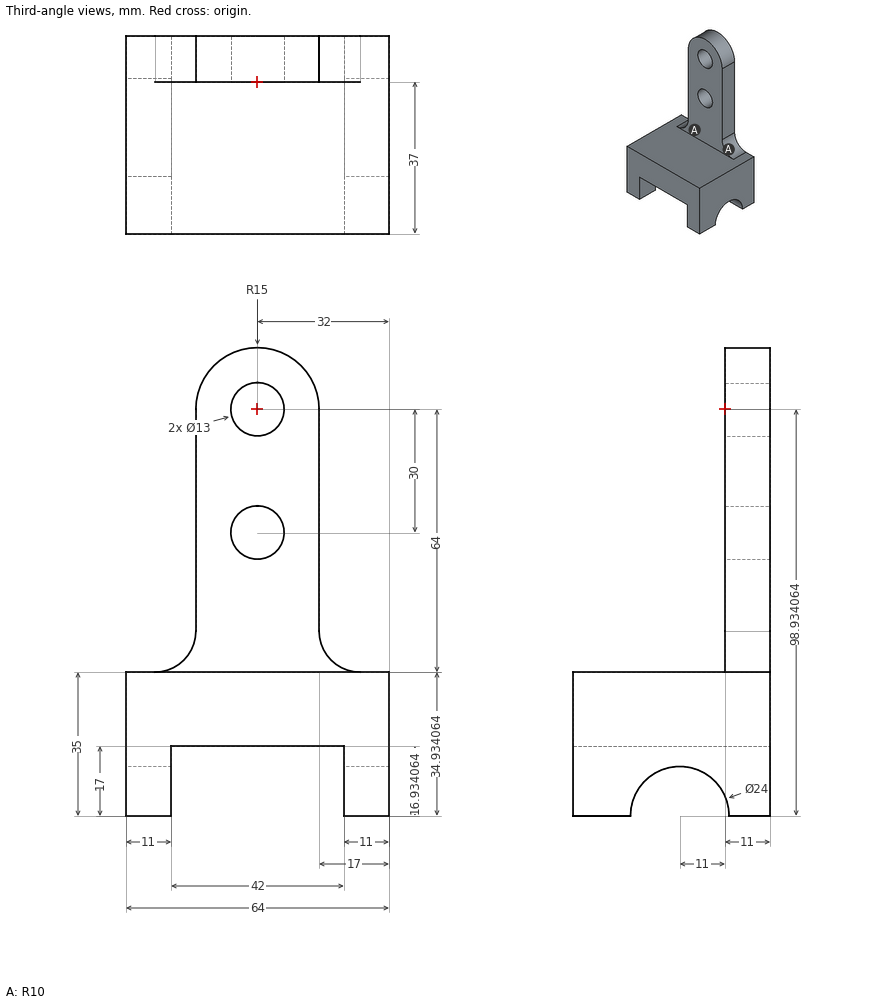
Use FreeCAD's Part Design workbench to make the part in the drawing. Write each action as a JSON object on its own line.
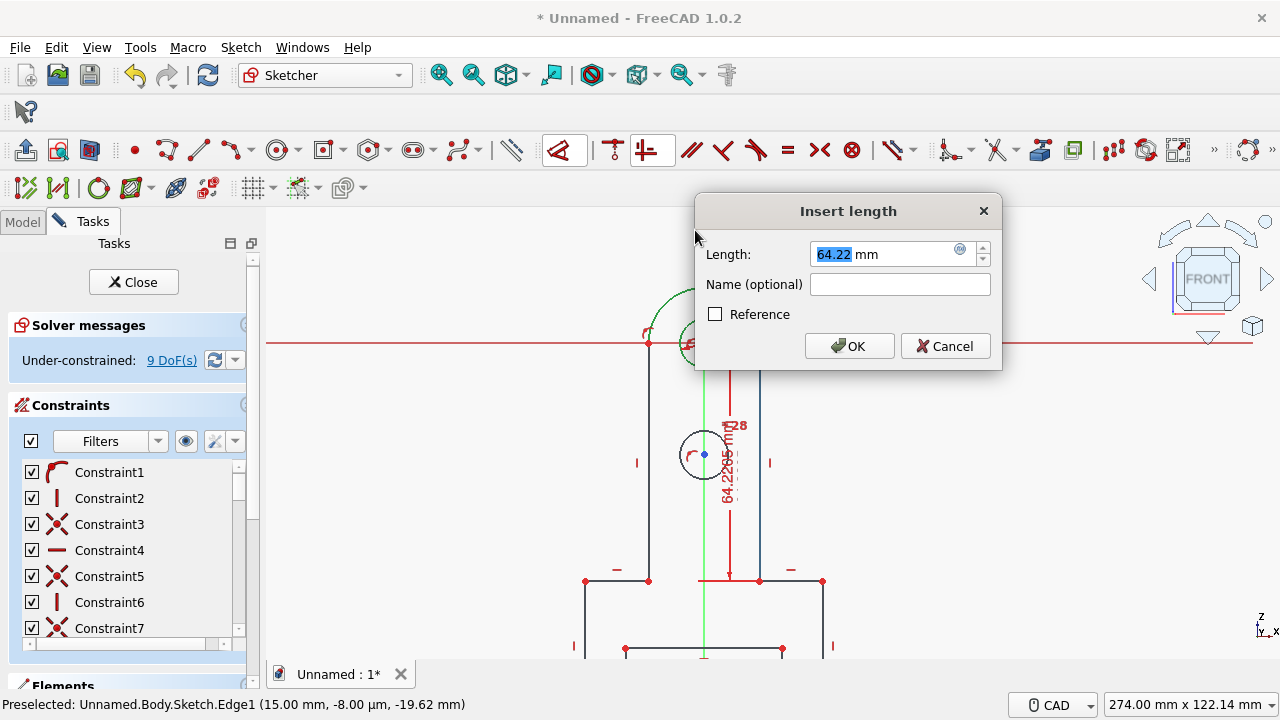
{"action": "type", "text": "64"}
{"action": "key", "text": "Return"}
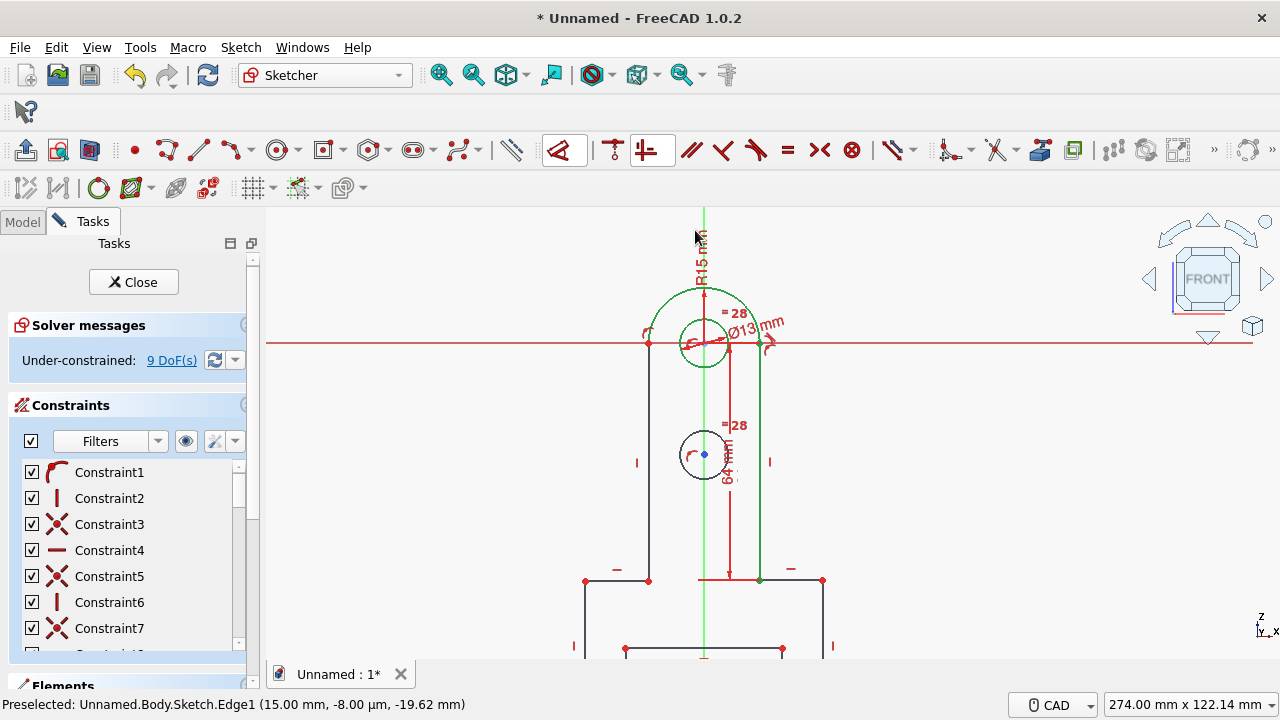
{"action": "left_click", "coordinate": [779, 580]}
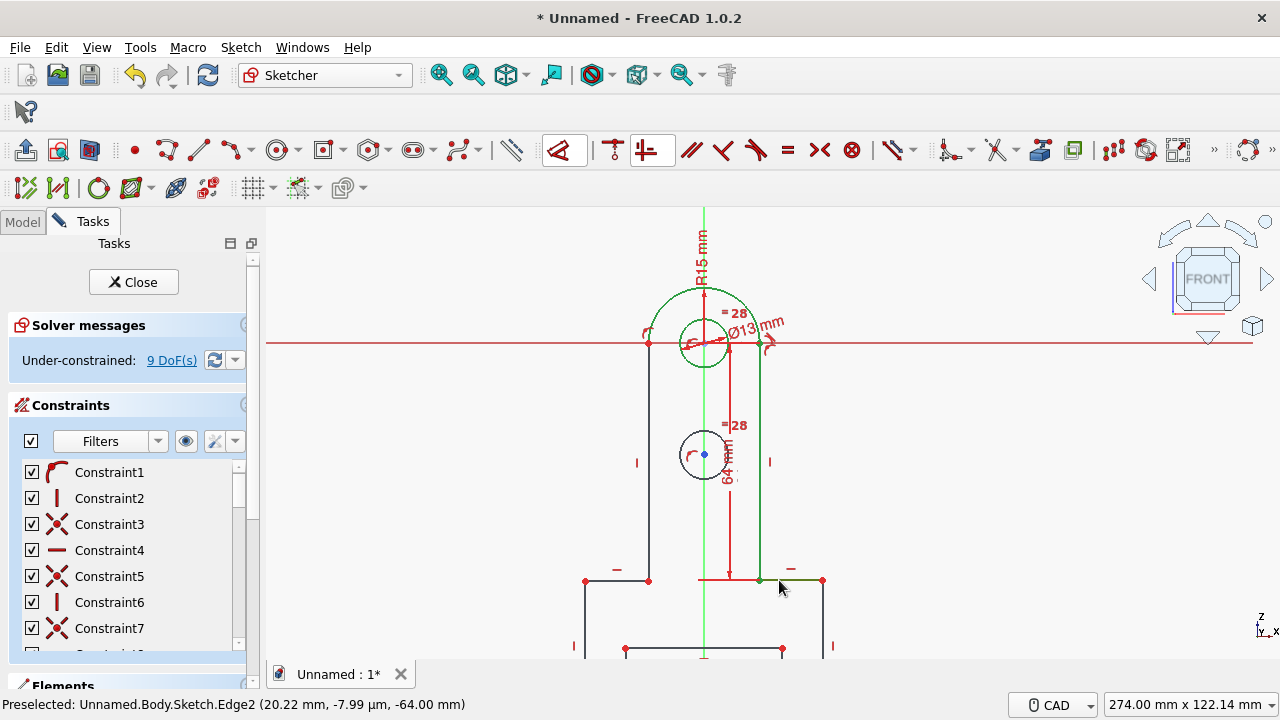
{"action": "left_click", "coordinate": [582, 150]}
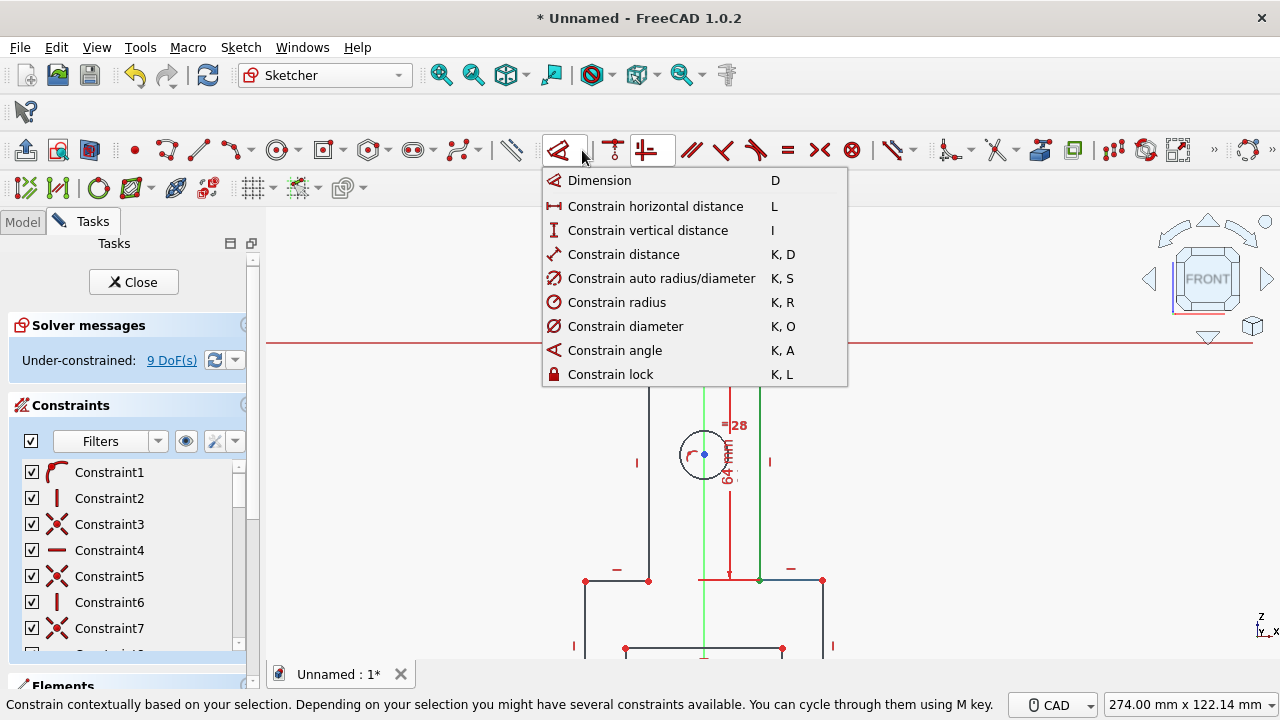
{"action": "left_click", "coordinate": [695, 206]}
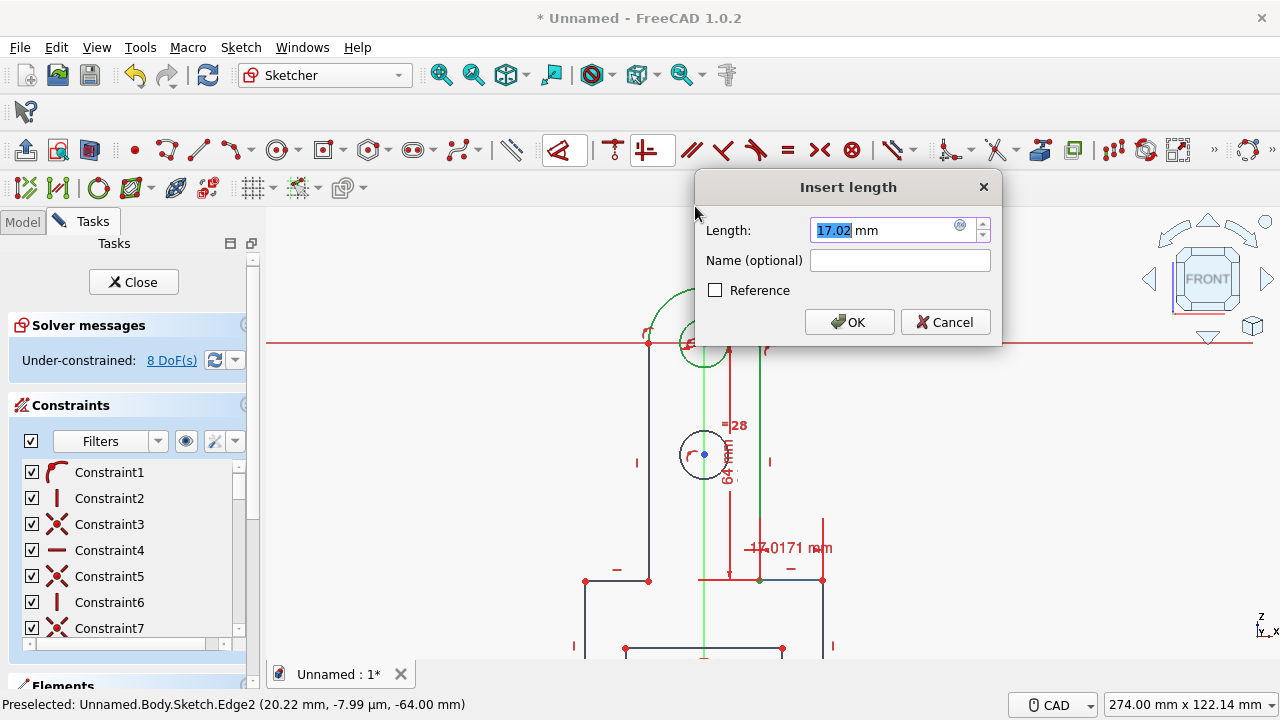
{"action": "type", "text": "17"}
{"action": "key", "text": "Return"}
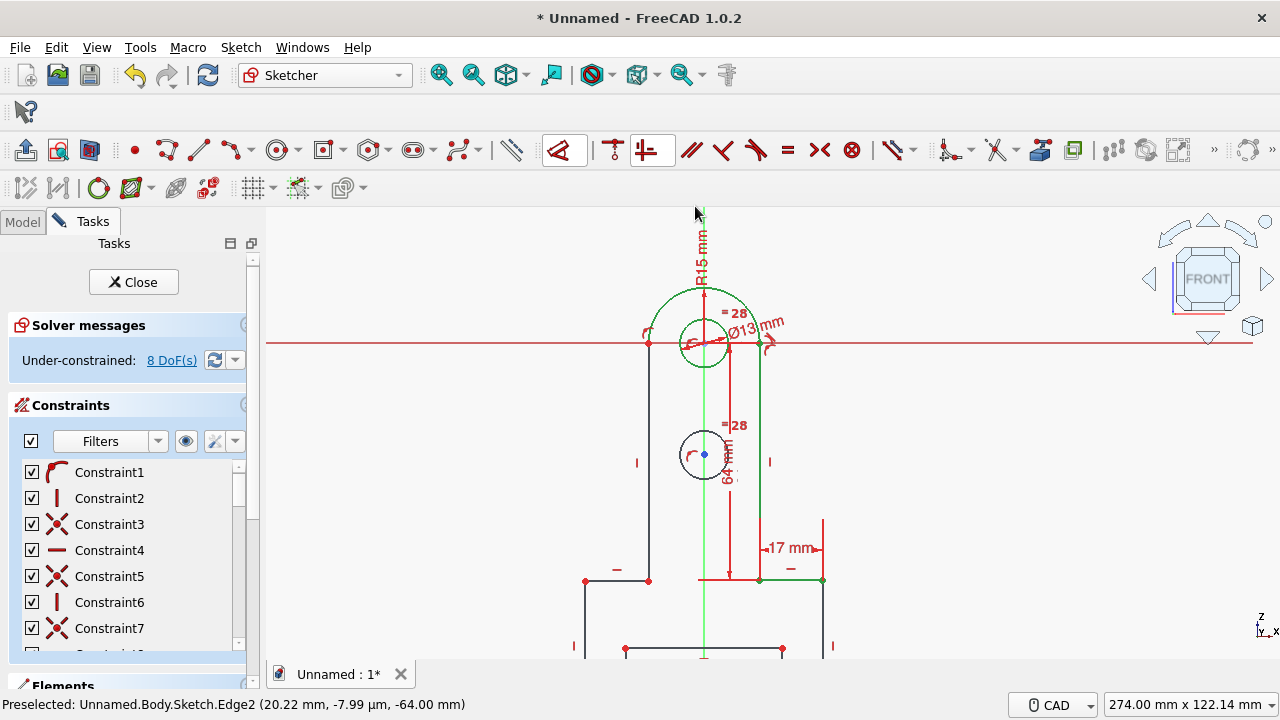
{"action": "scroll", "coordinate": [705, 299], "scroll_direction": "down", "scroll_amount": 2}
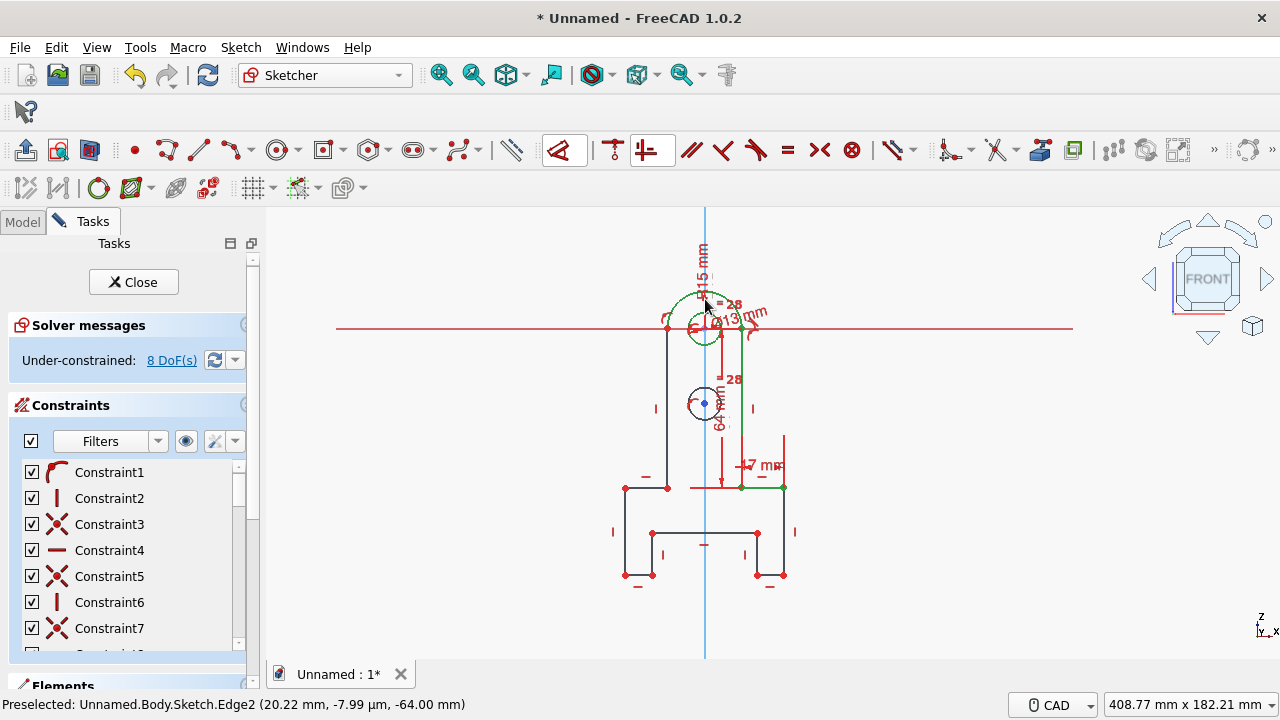
{"action": "scroll", "coordinate": [776, 575], "scroll_direction": "up", "scroll_amount": 3}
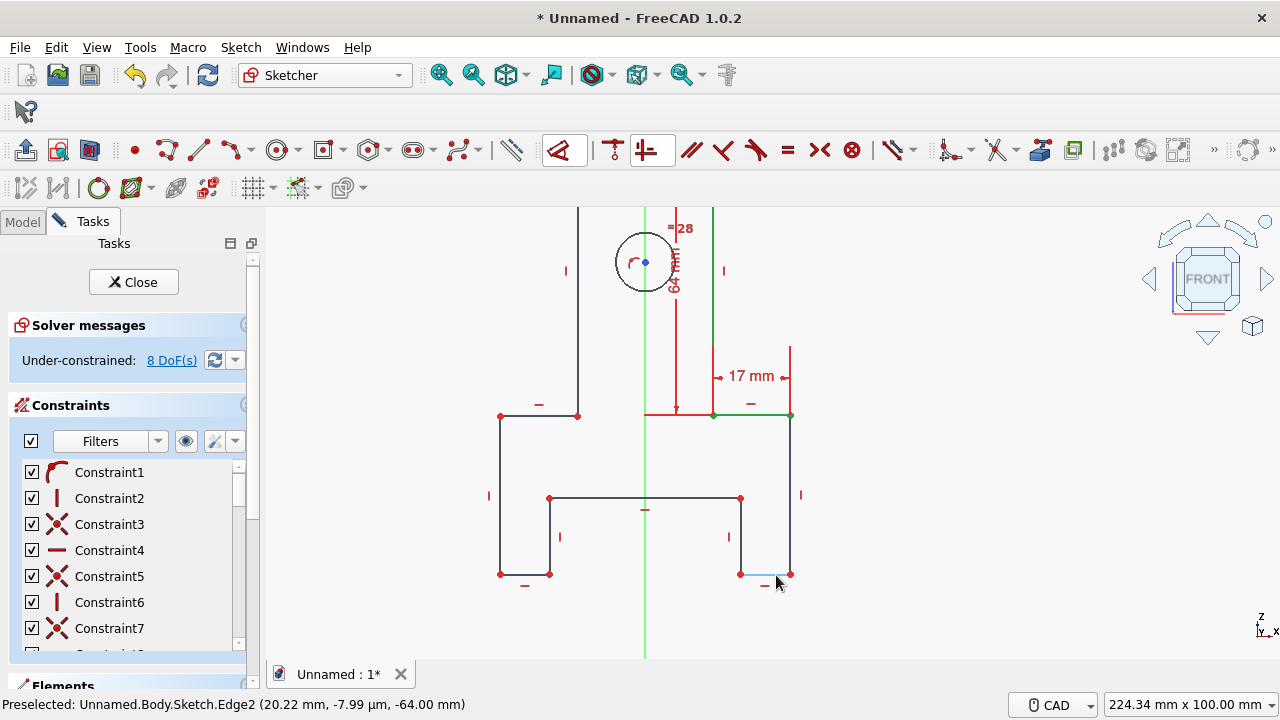
{"action": "left_click", "coordinate": [775, 575]}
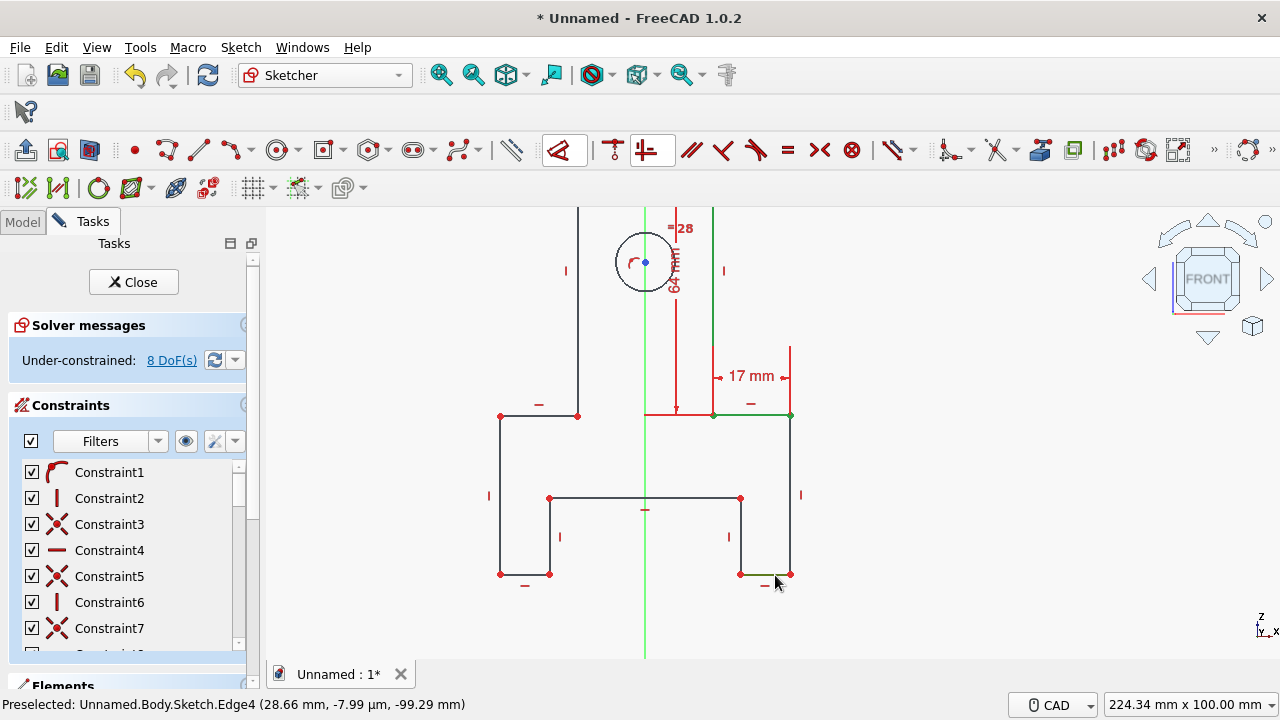
{"action": "key", "text": "l"}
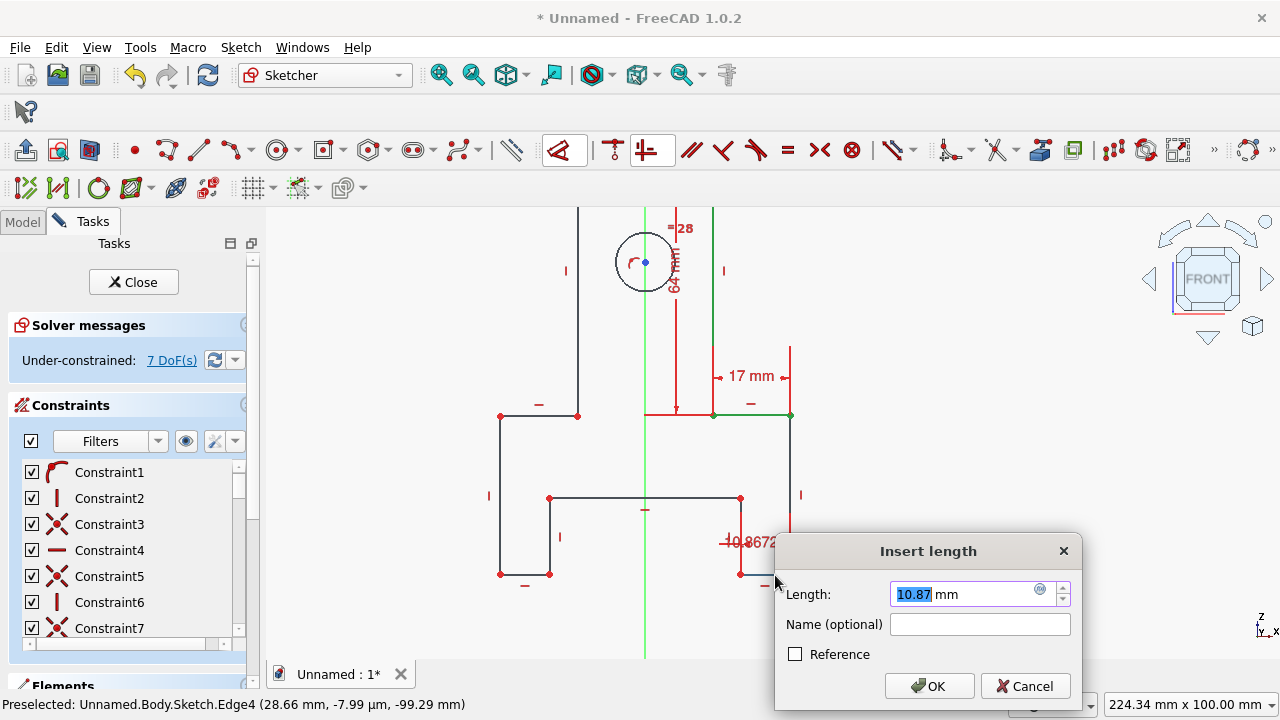
{"action": "type", "text": "11"}
{"action": "key", "text": "Return"}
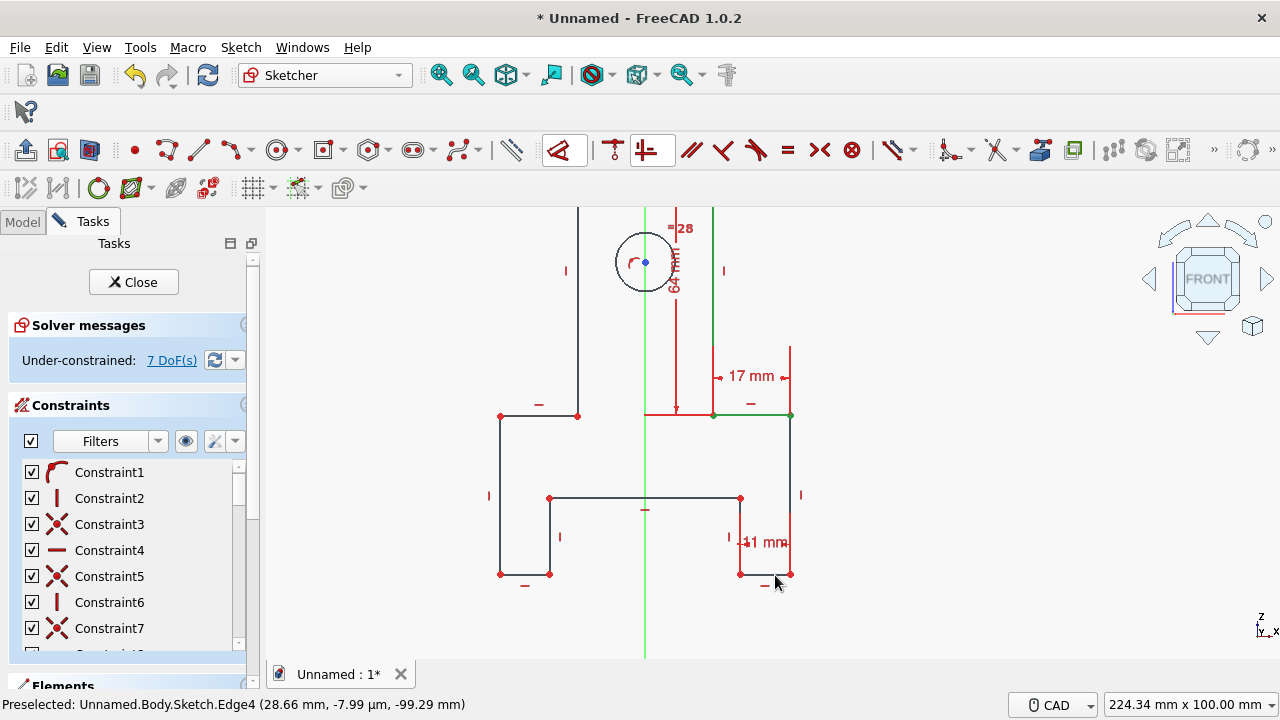
{"action": "left_click", "coordinate": [683, 498]}